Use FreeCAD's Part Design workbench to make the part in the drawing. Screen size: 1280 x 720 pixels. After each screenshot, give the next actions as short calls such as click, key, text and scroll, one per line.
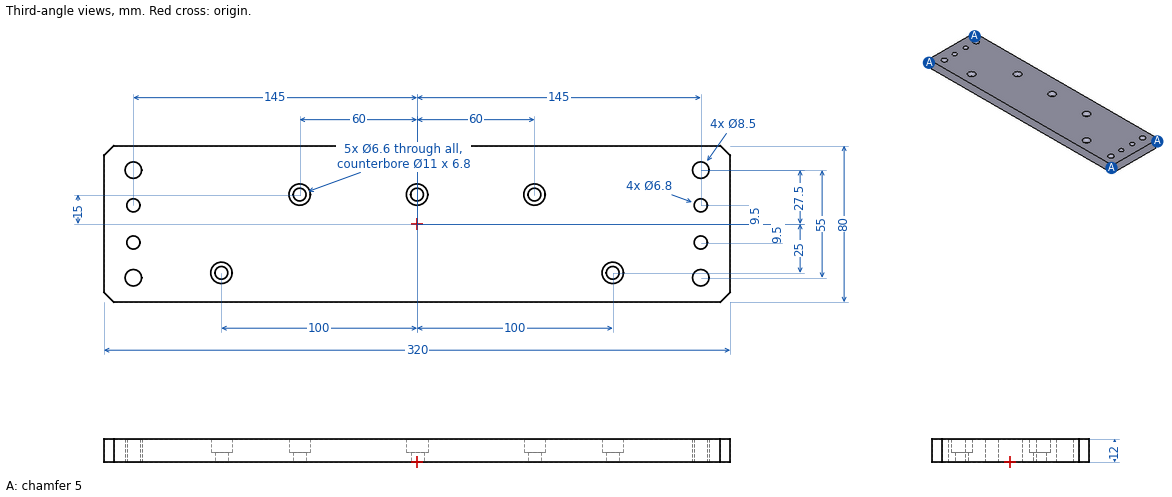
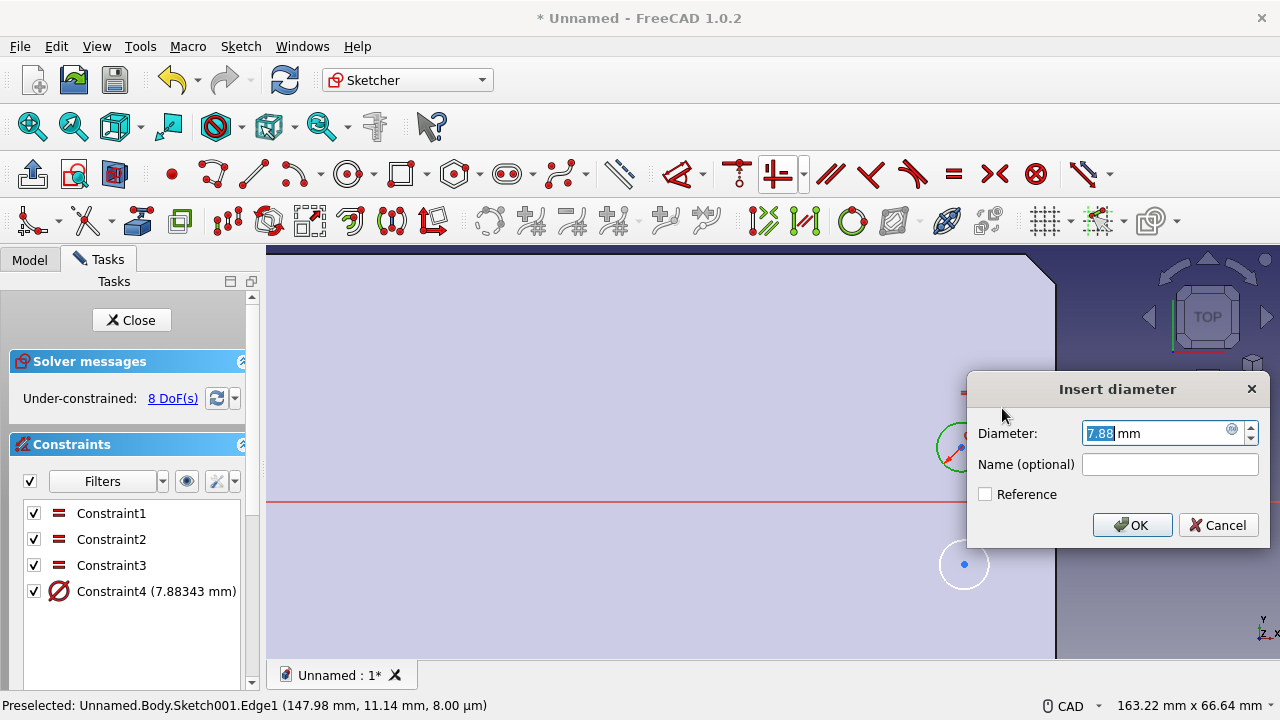
text(6.8)
key(Return)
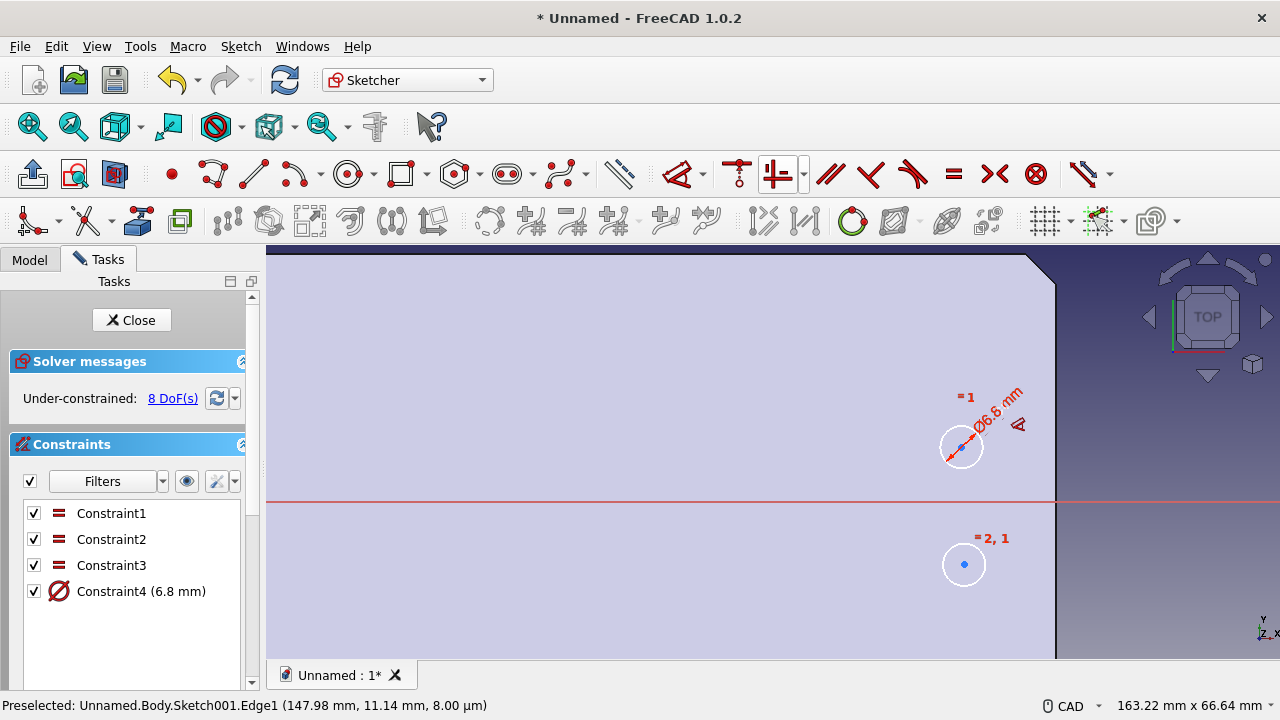
click(962, 447)
click(628, 413)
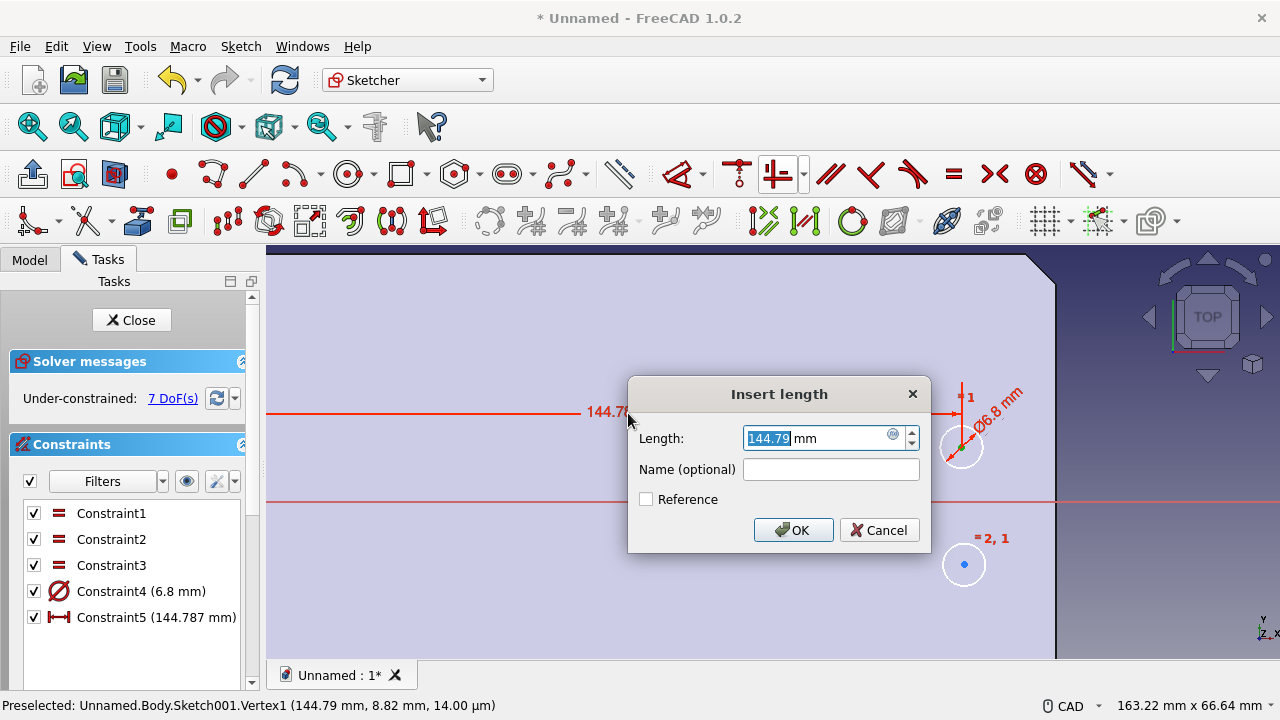
text(145)
key(Return)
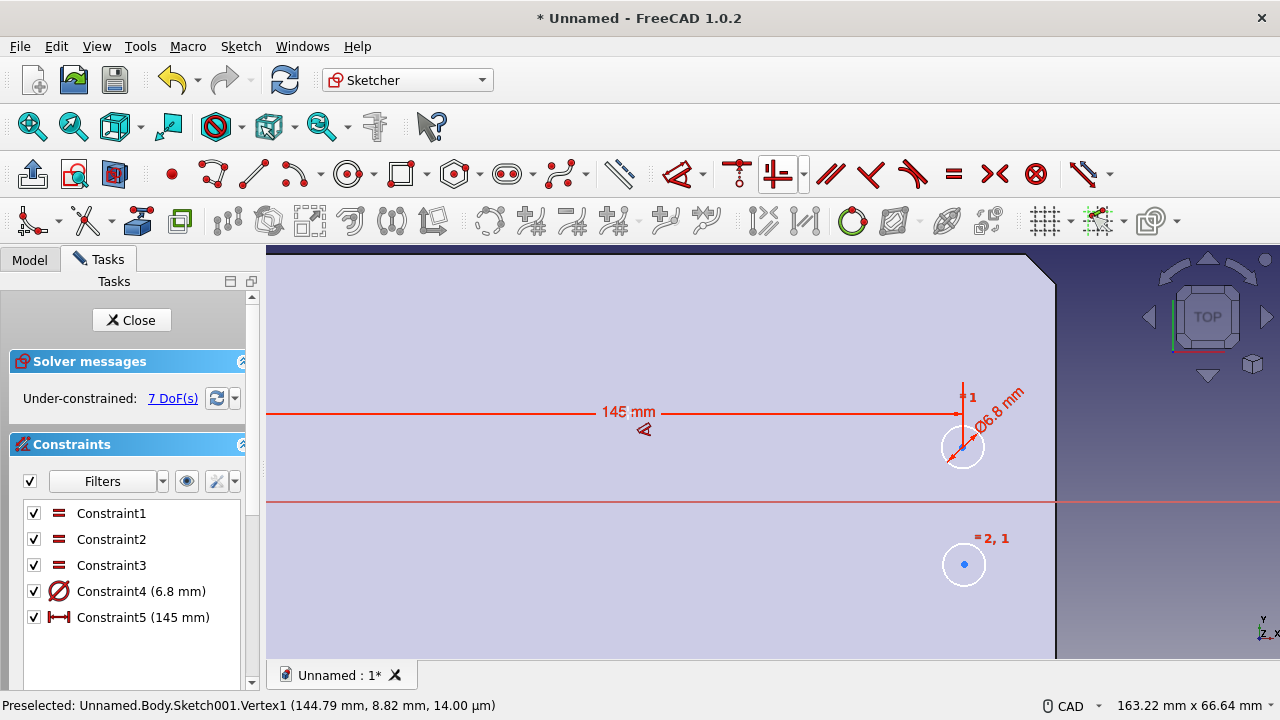
click(963, 447)
click(997, 475)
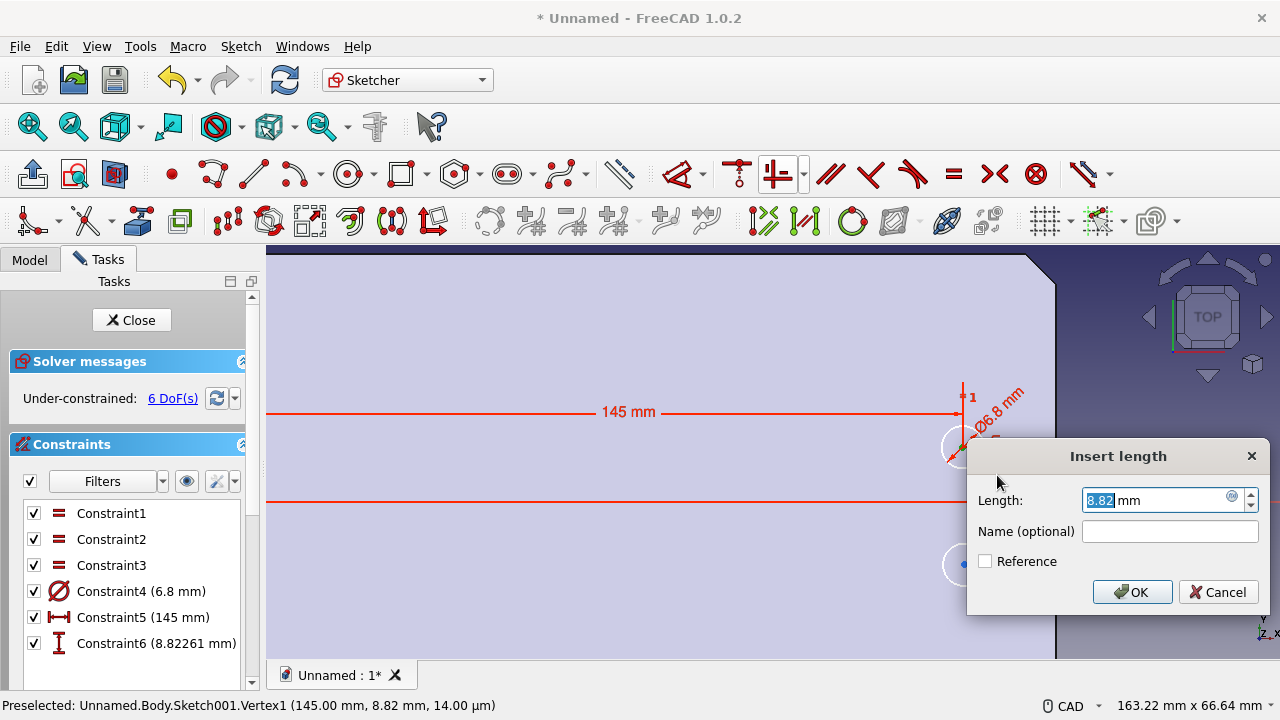
text(9.5)
key(Return)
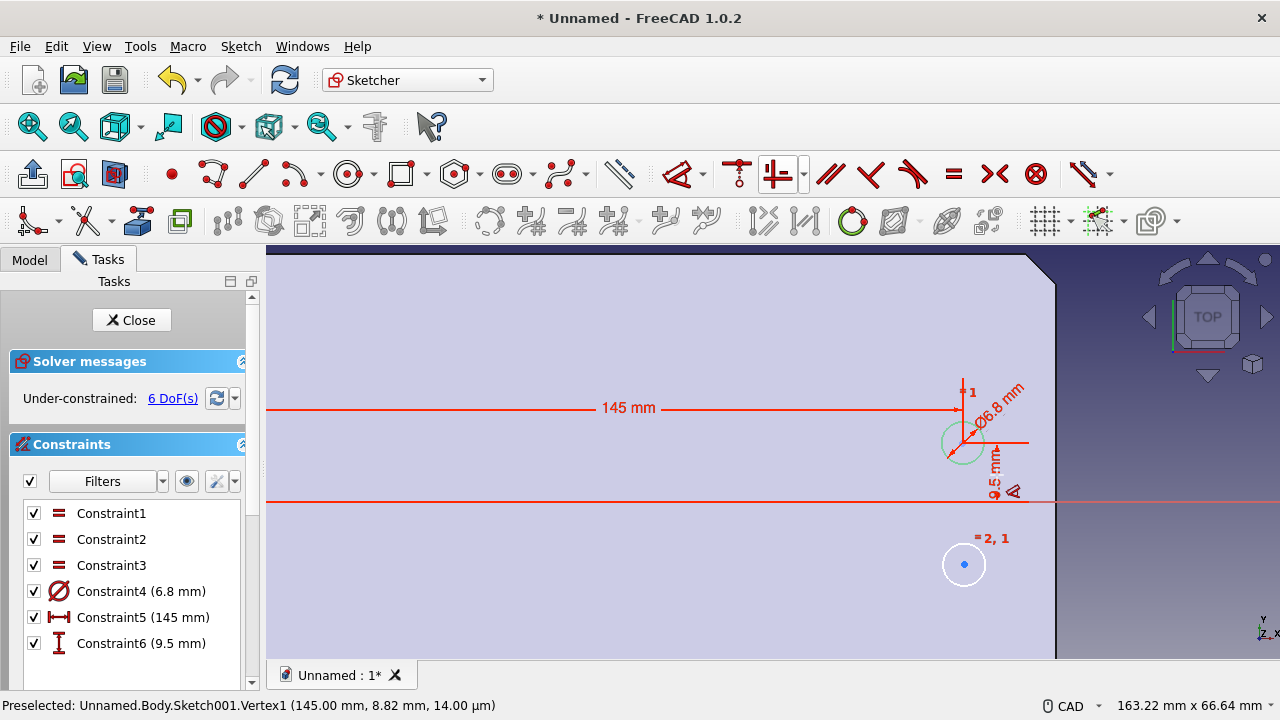
click(964, 565)
click(629, 599)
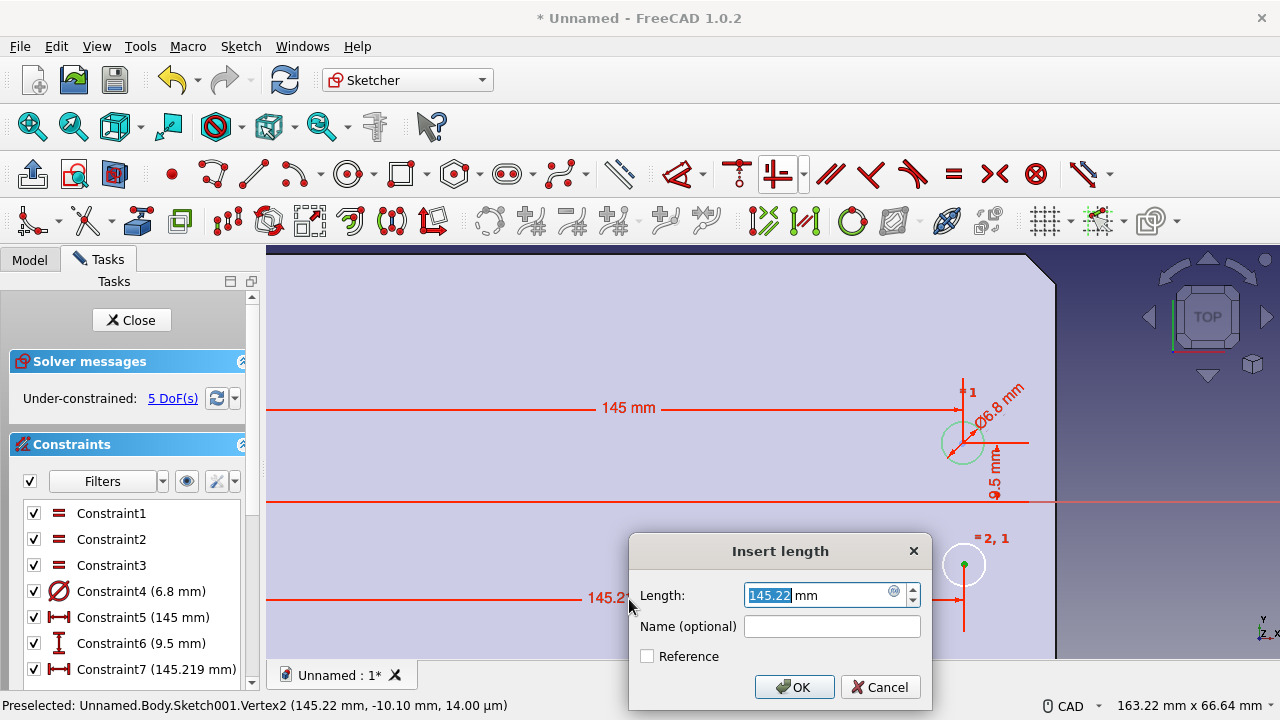
text(145)
key(Return)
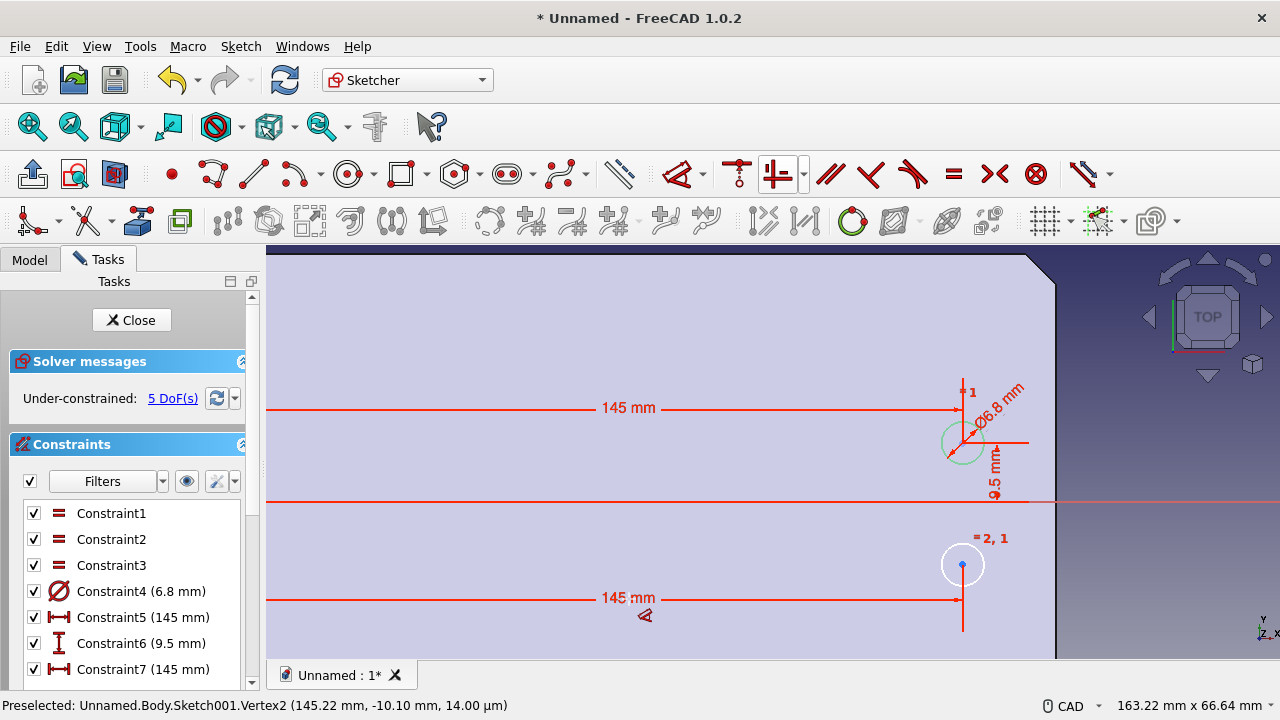
click(963, 565)
click(997, 533)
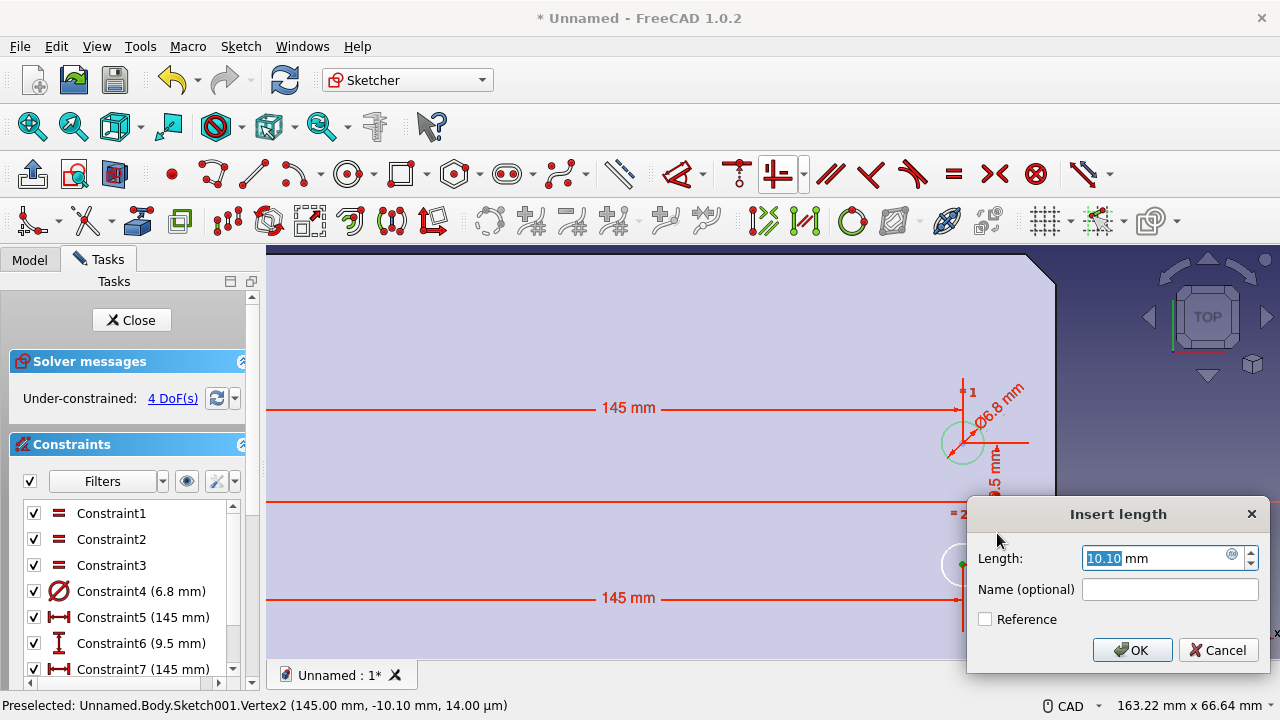
text(9.5)
key(Return)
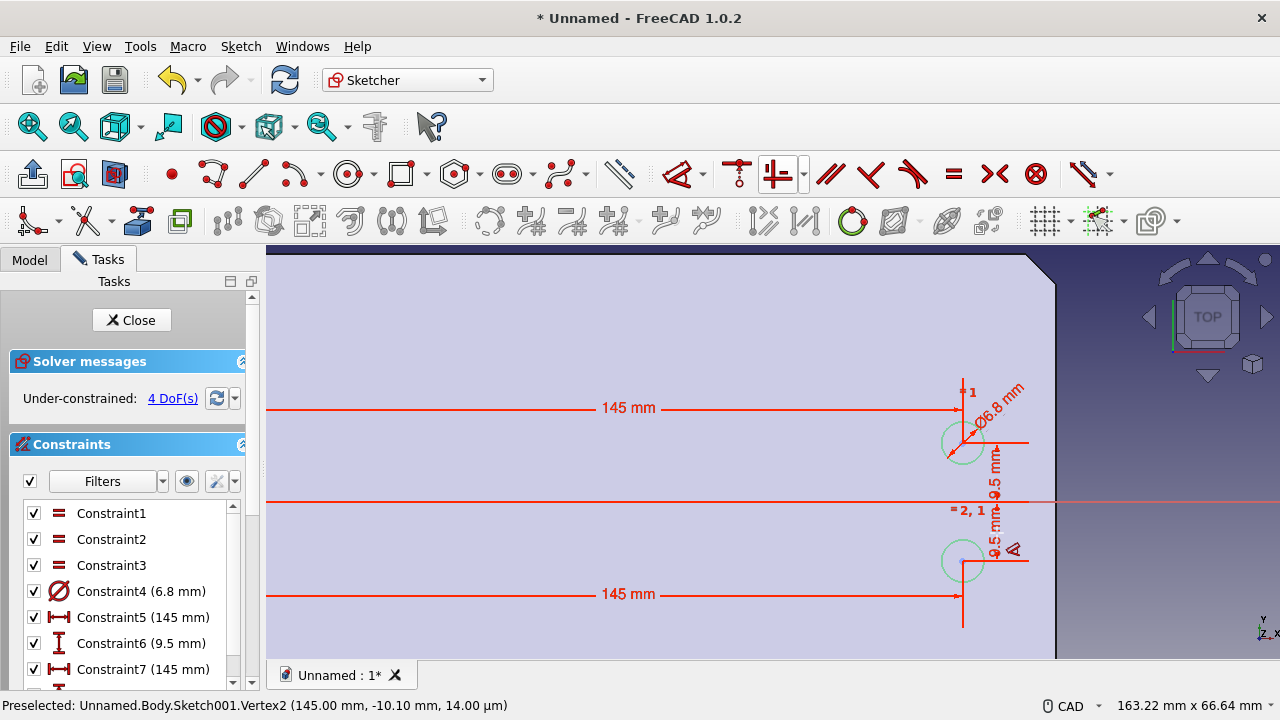
scroll(981, 430, down, 6)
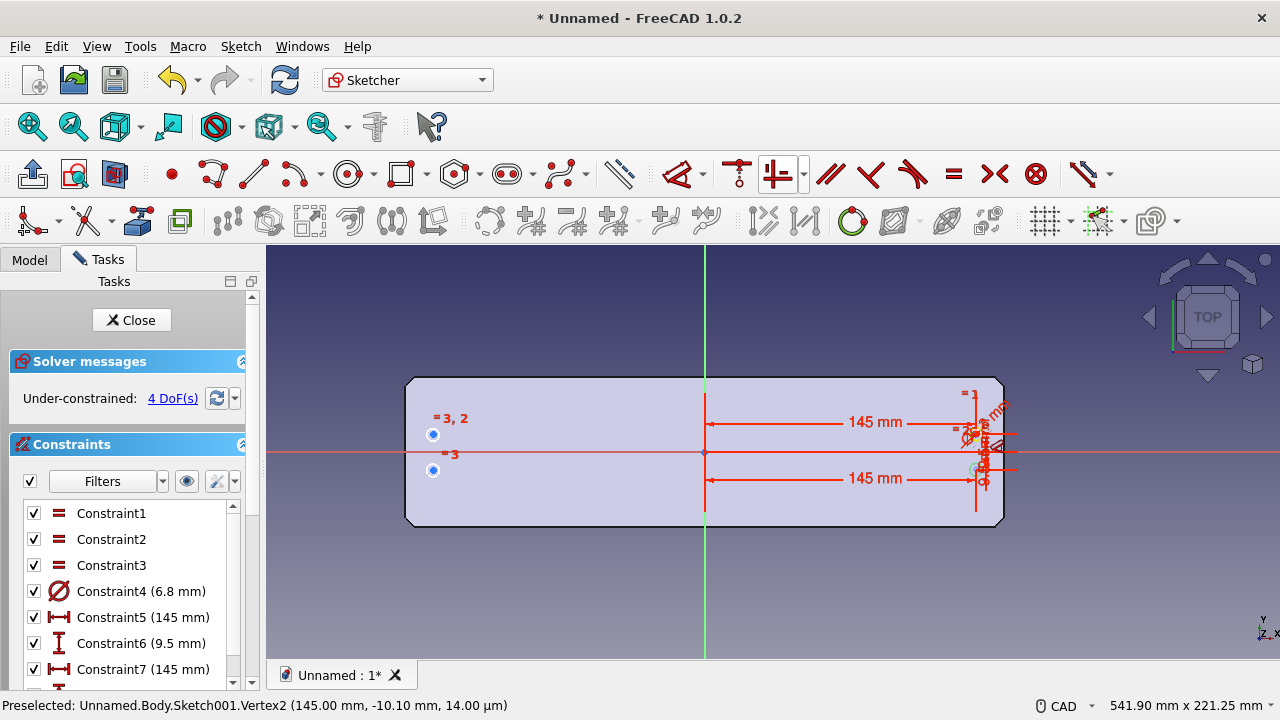
click(433, 435)
click(569, 401)